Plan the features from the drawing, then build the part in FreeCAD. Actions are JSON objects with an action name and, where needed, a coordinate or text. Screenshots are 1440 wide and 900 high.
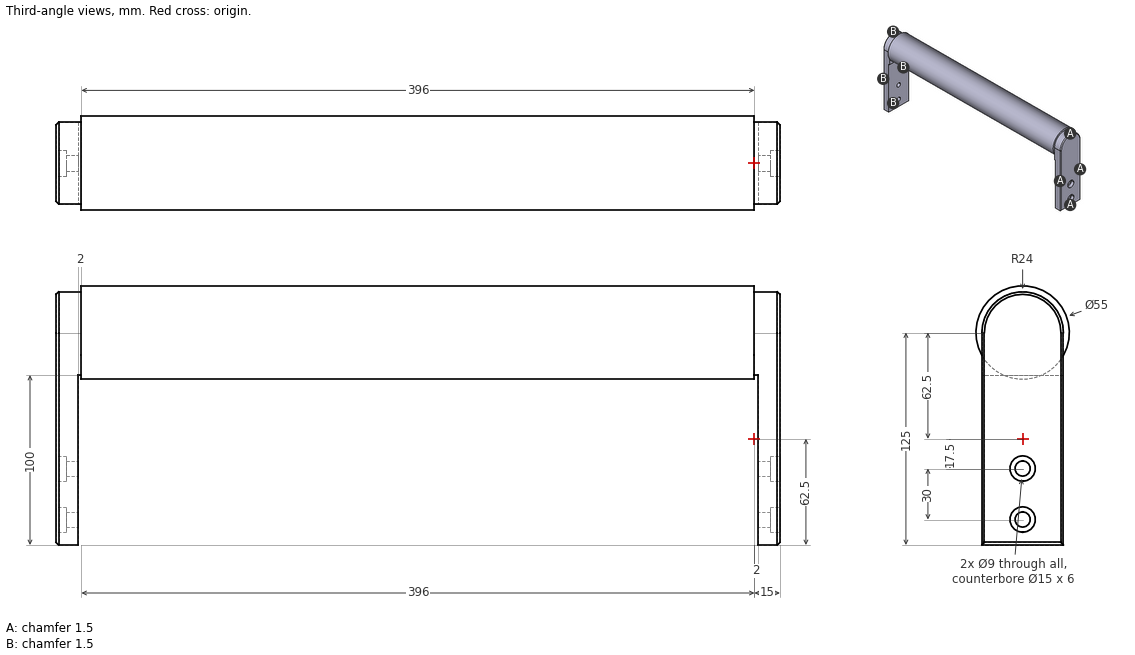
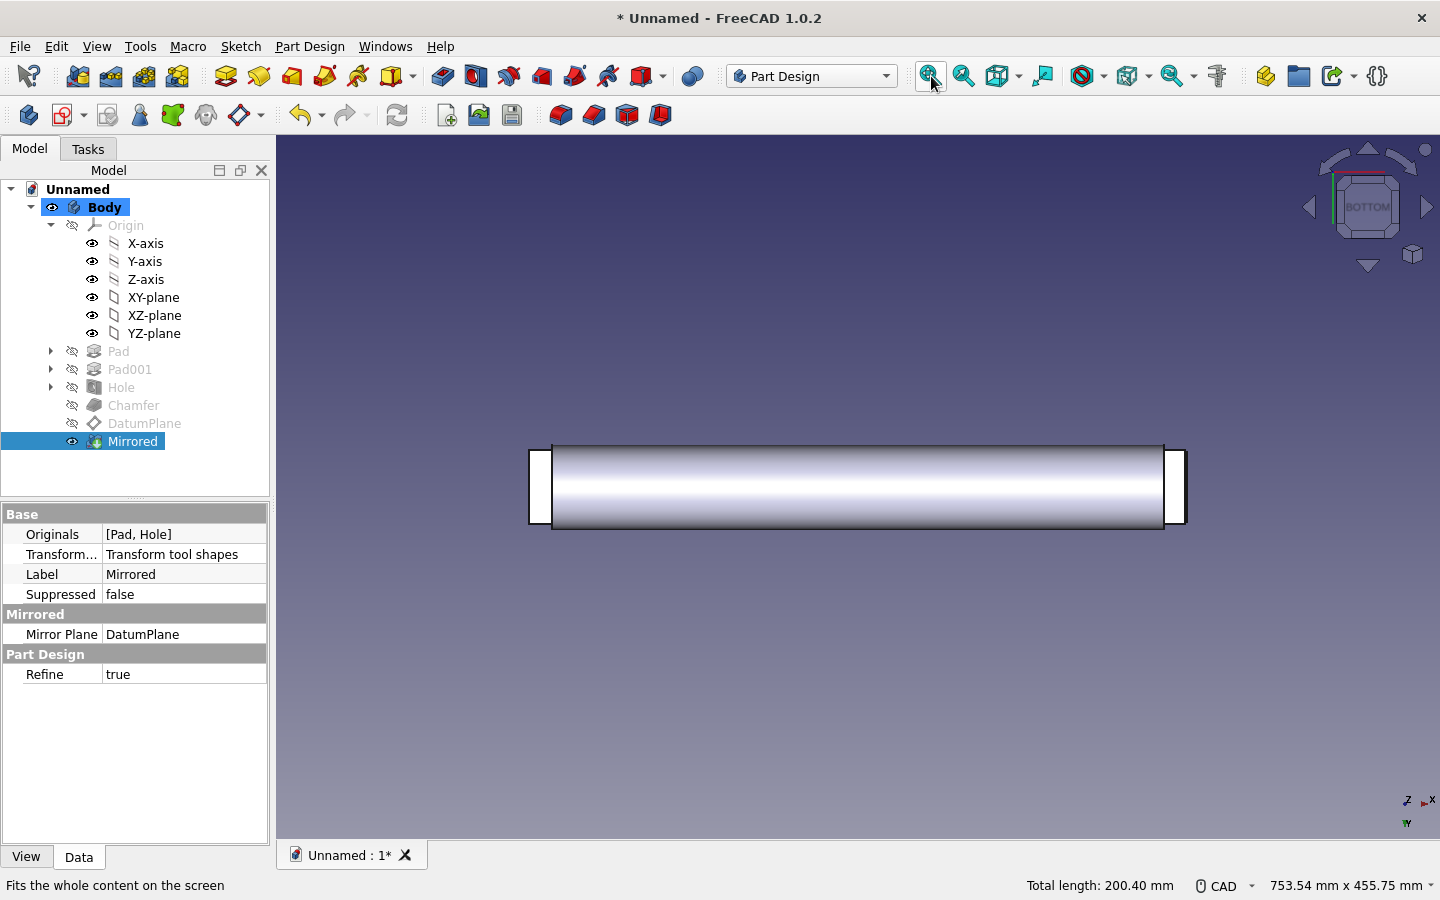
{"action": "left_click", "coordinate": [529, 486], "text": "ctrl"}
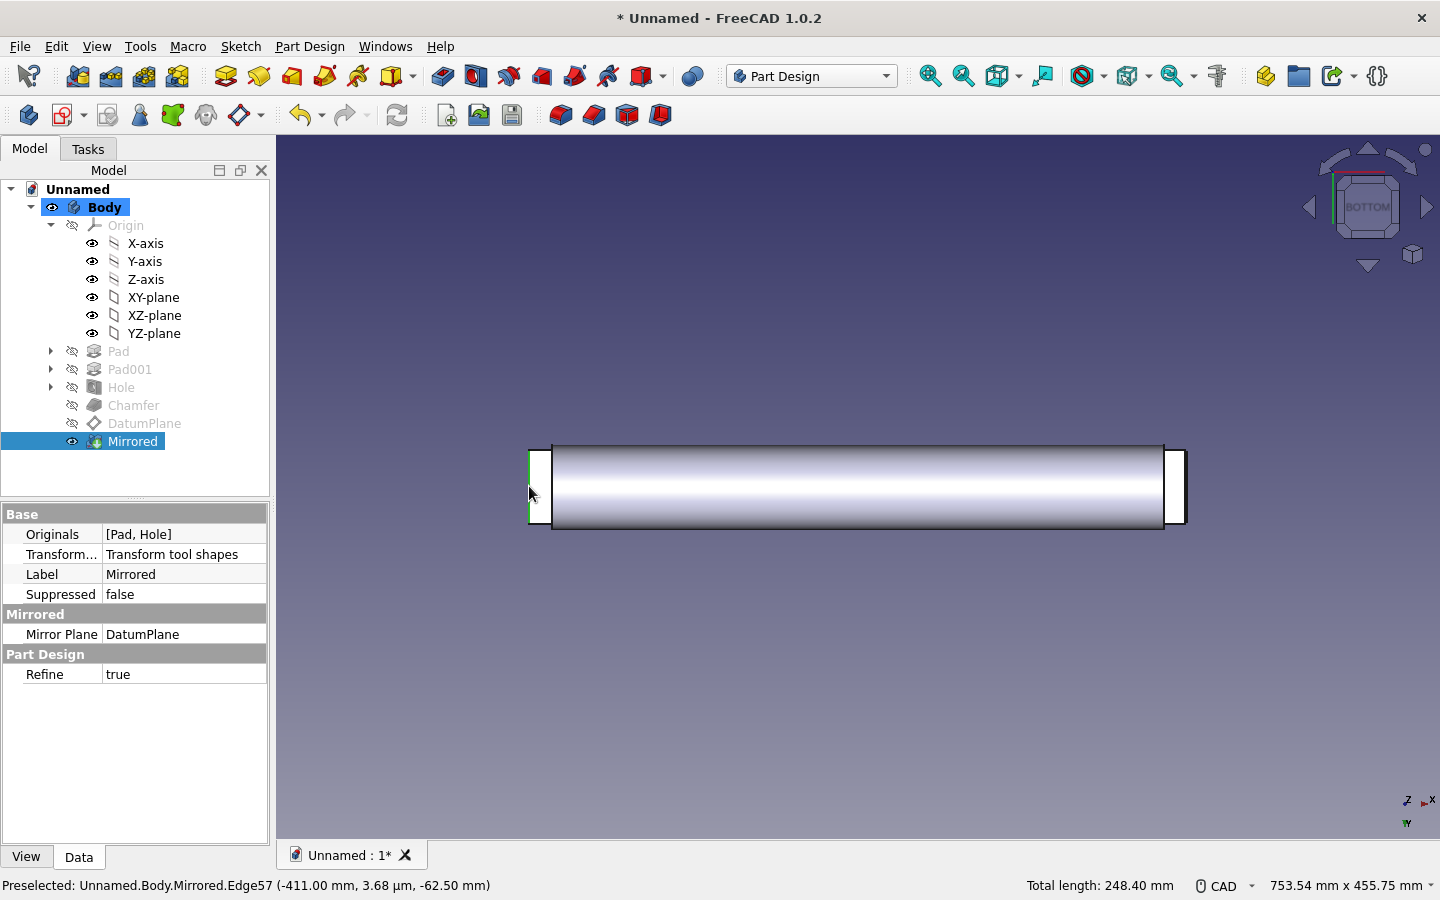
{"action": "key", "text": "4"}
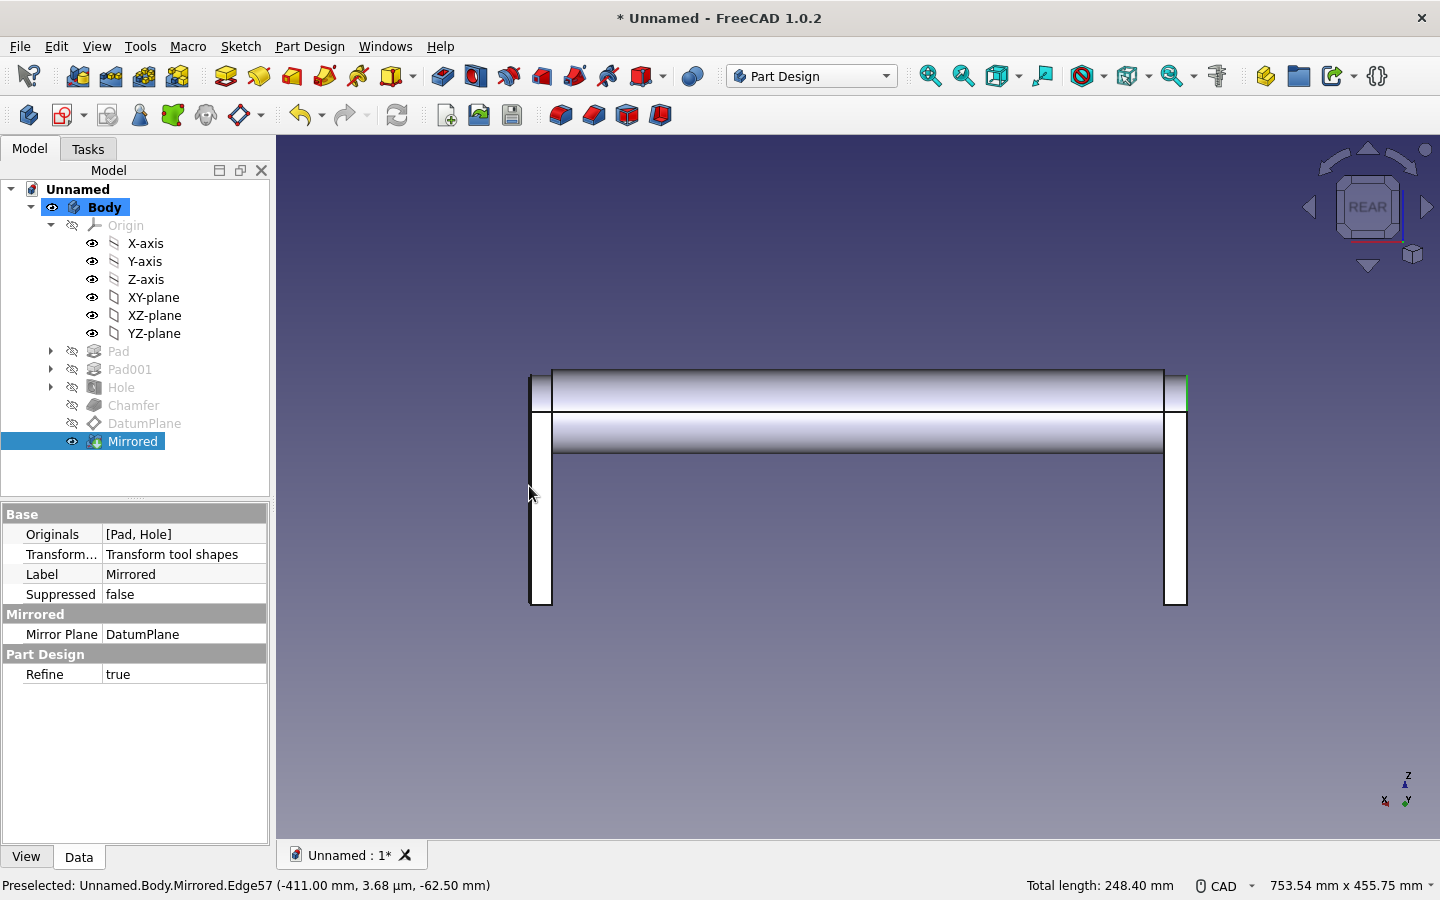
{"action": "left_click", "coordinate": [1187, 507], "text": "ctrl"}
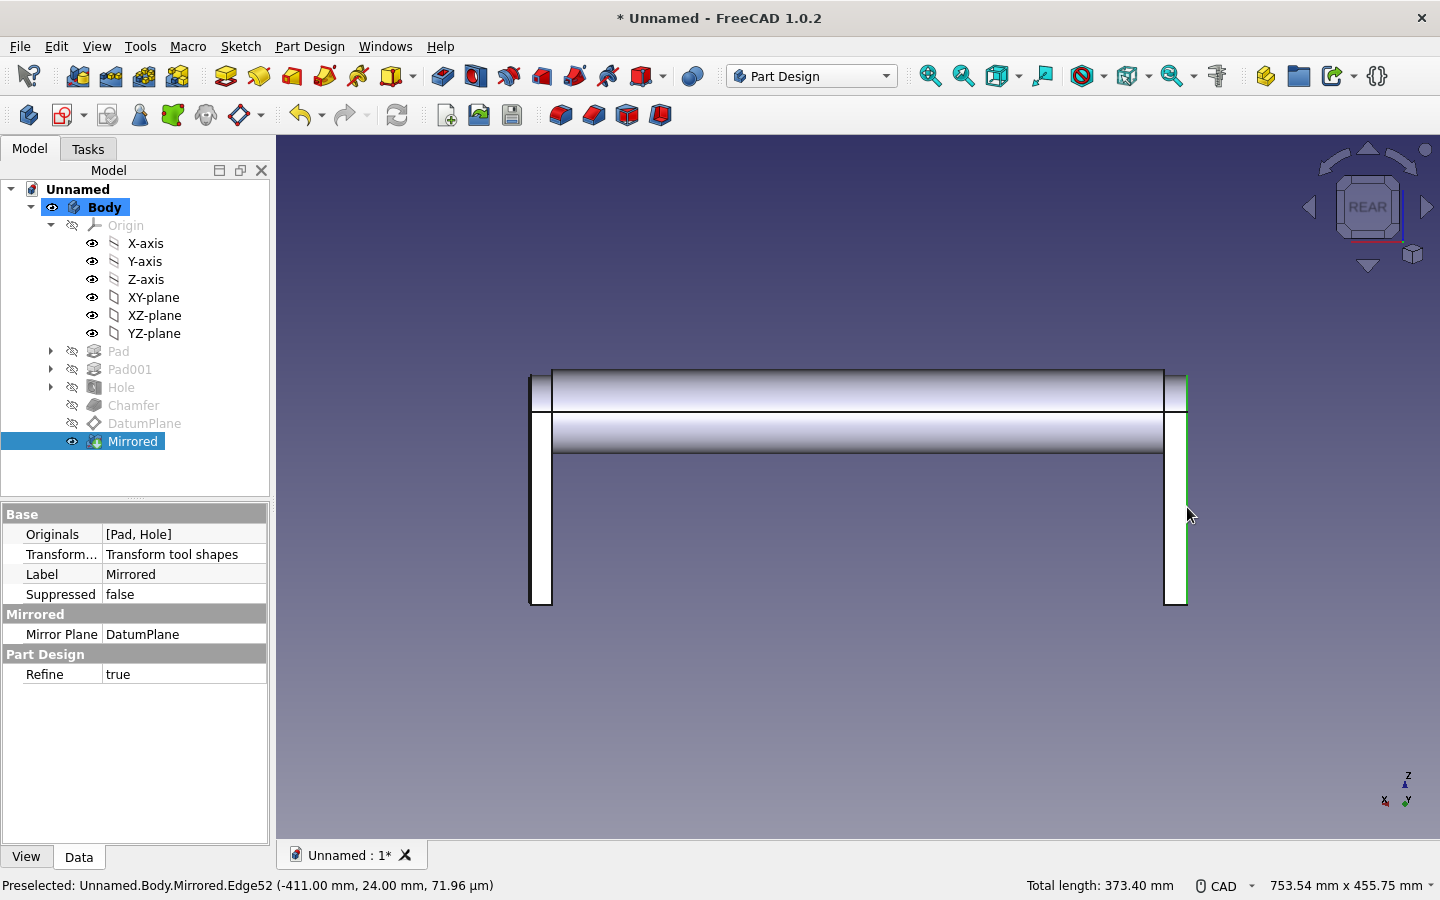
{"action": "left_click", "coordinate": [594, 116]}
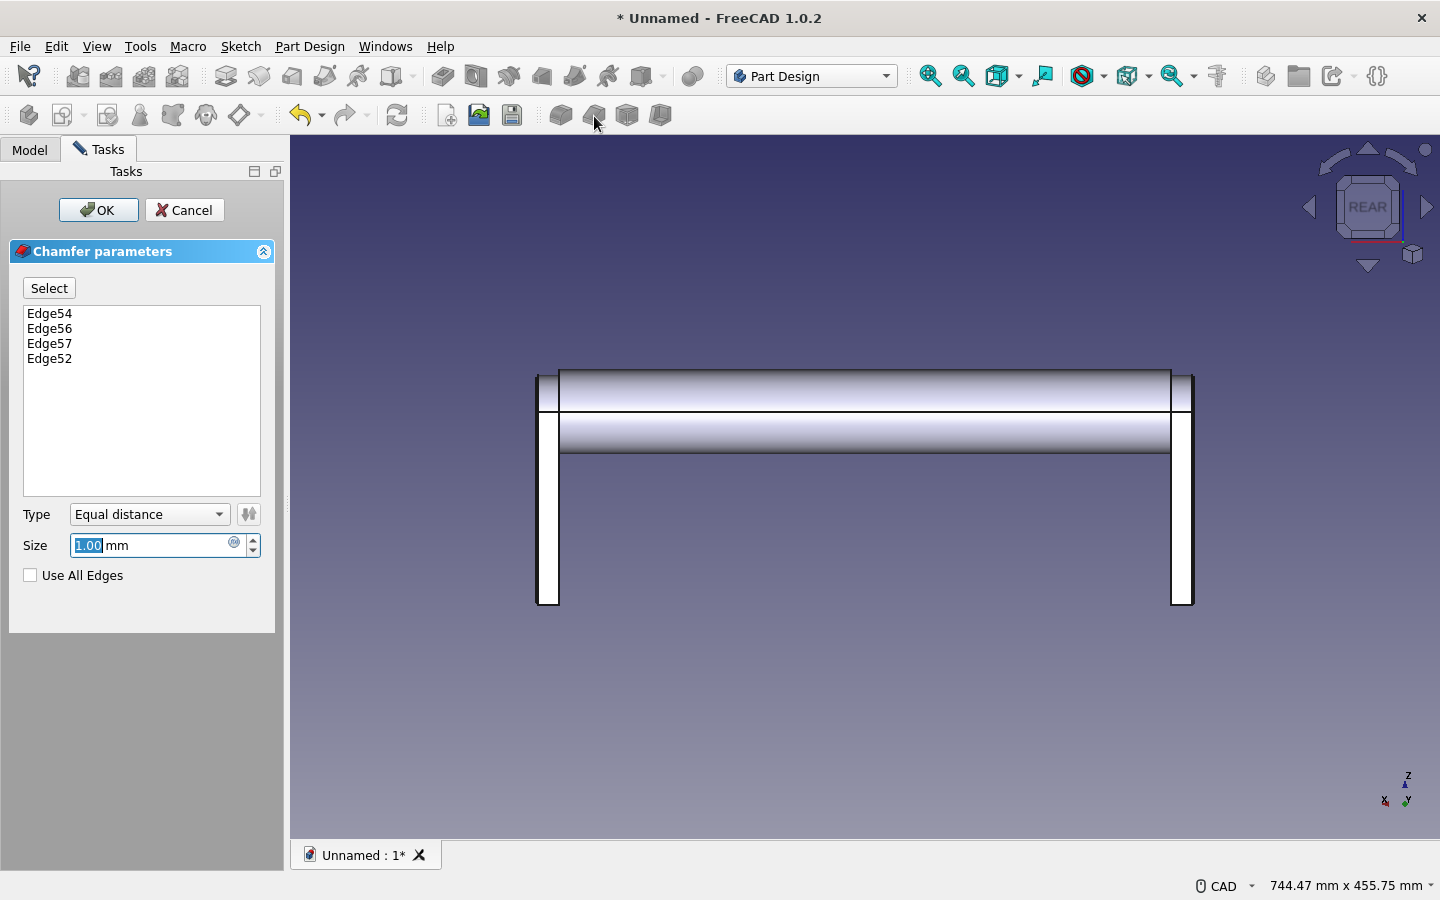
{"action": "type", "text": "1.5"}
{"action": "key", "text": "Tab"}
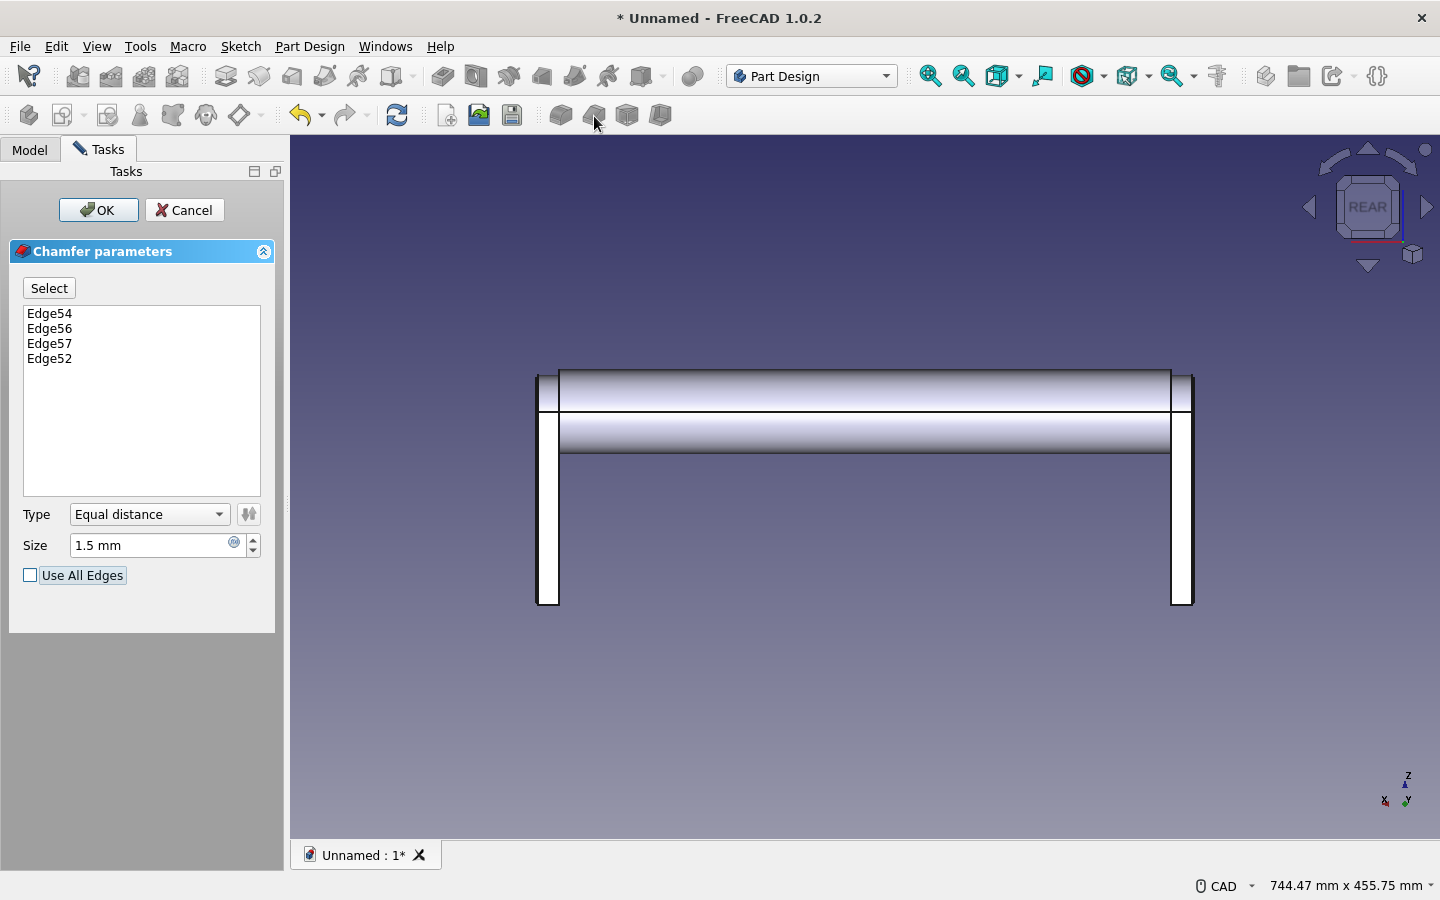
{"action": "left_click", "coordinate": [99, 210]}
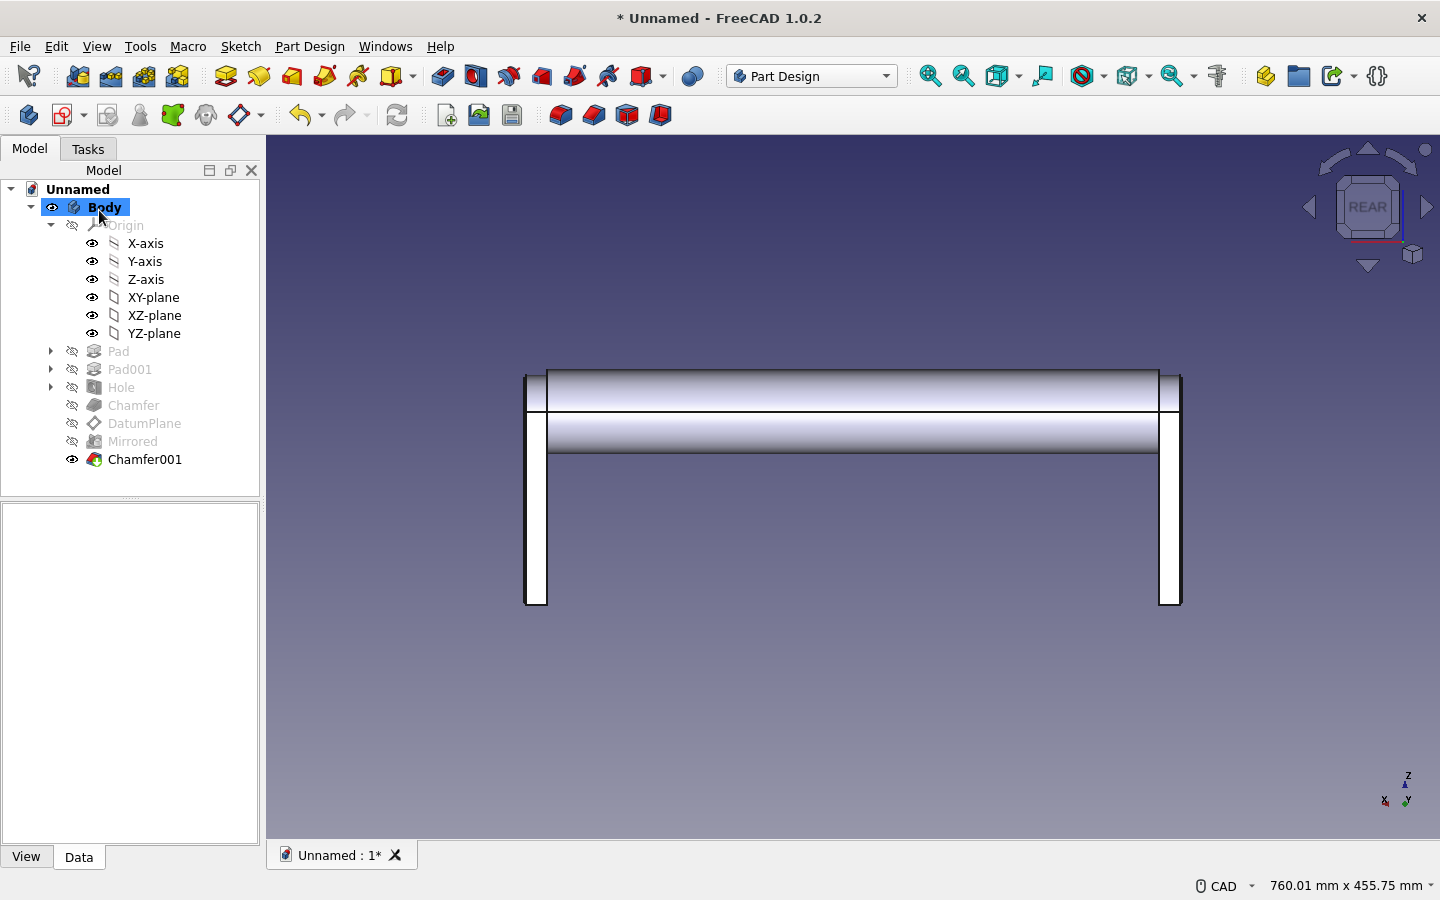
{"action": "left_click", "coordinate": [1169, 590]}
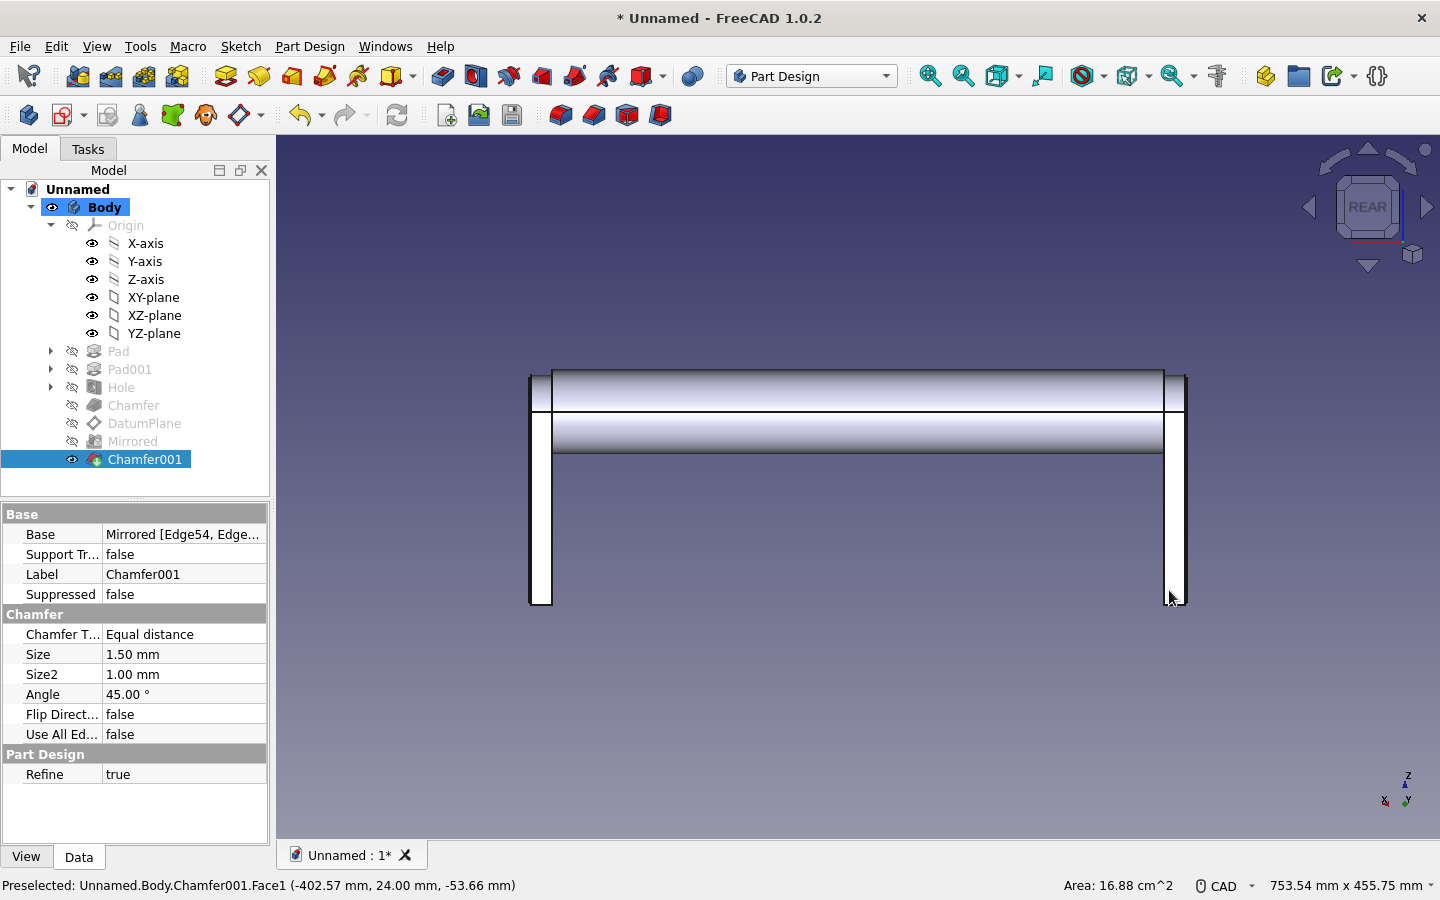
{"action": "left_click", "coordinate": [62, 116]}